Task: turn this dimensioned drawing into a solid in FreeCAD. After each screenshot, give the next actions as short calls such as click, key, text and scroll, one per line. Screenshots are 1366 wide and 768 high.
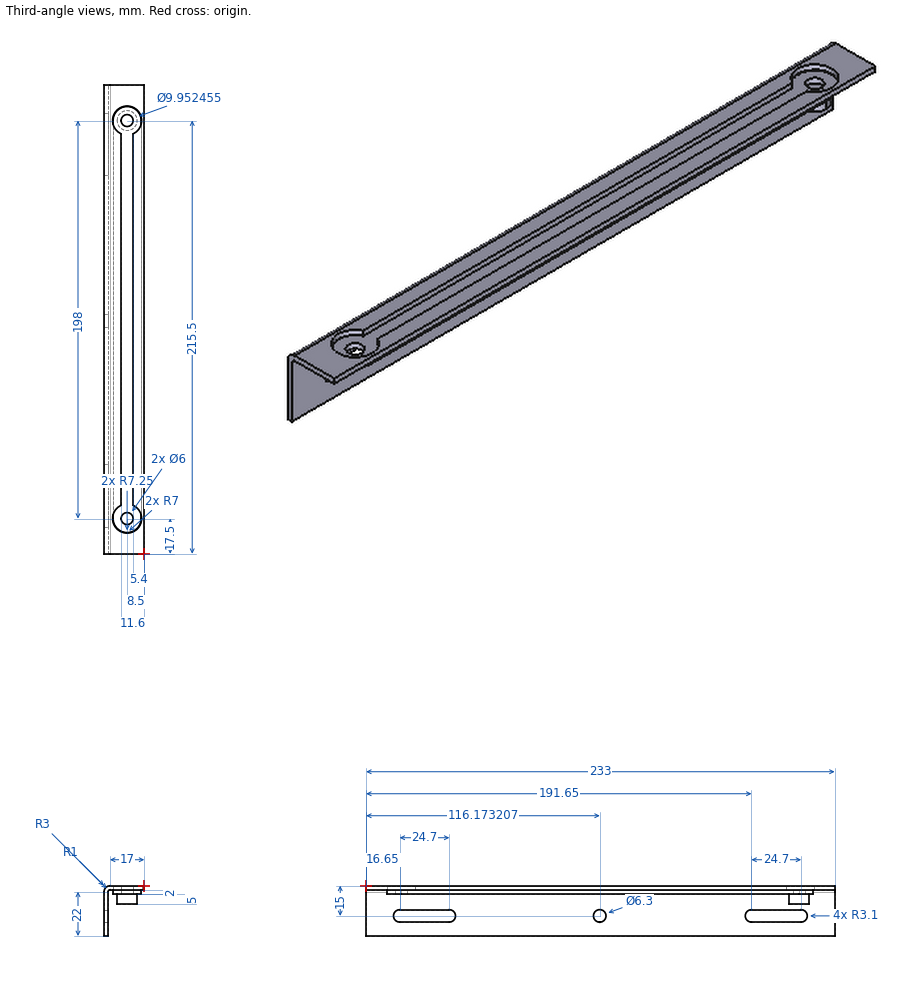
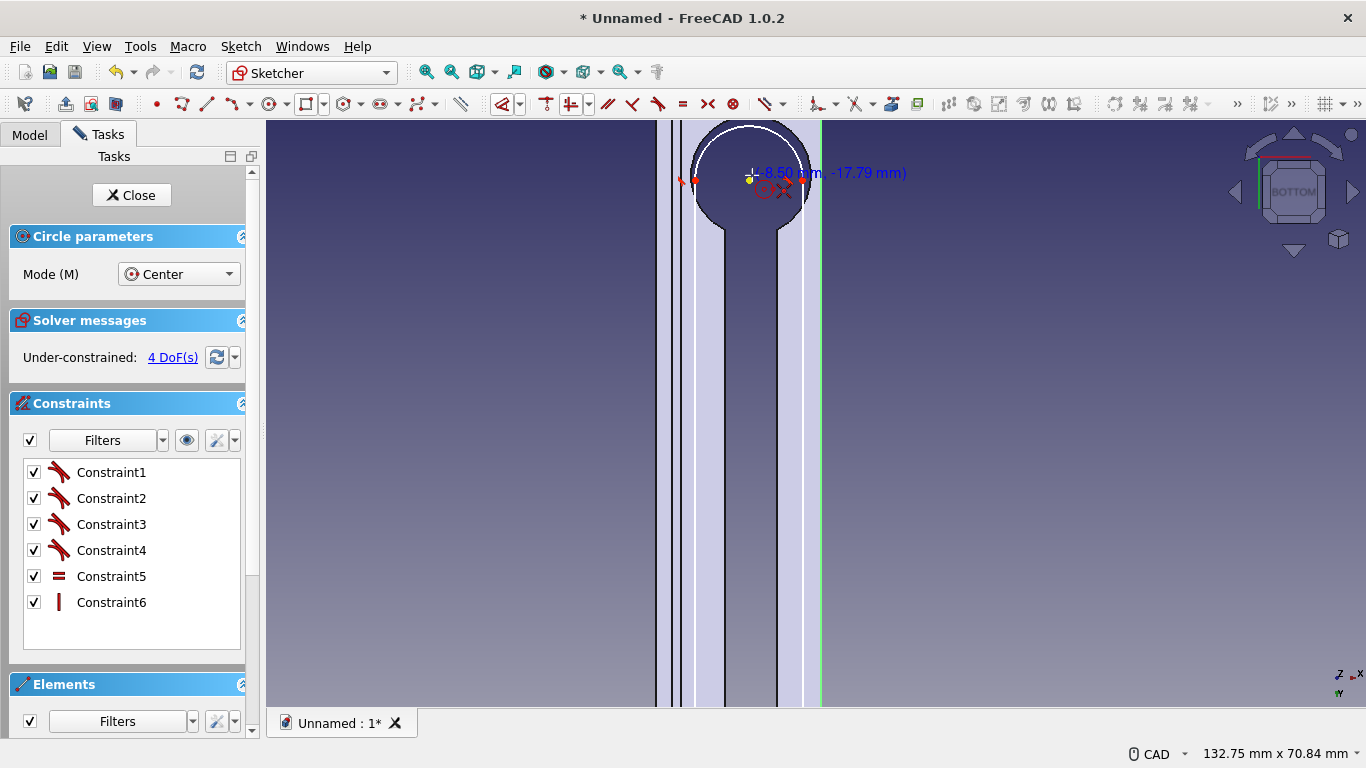
scroll(745, 277, down, 8)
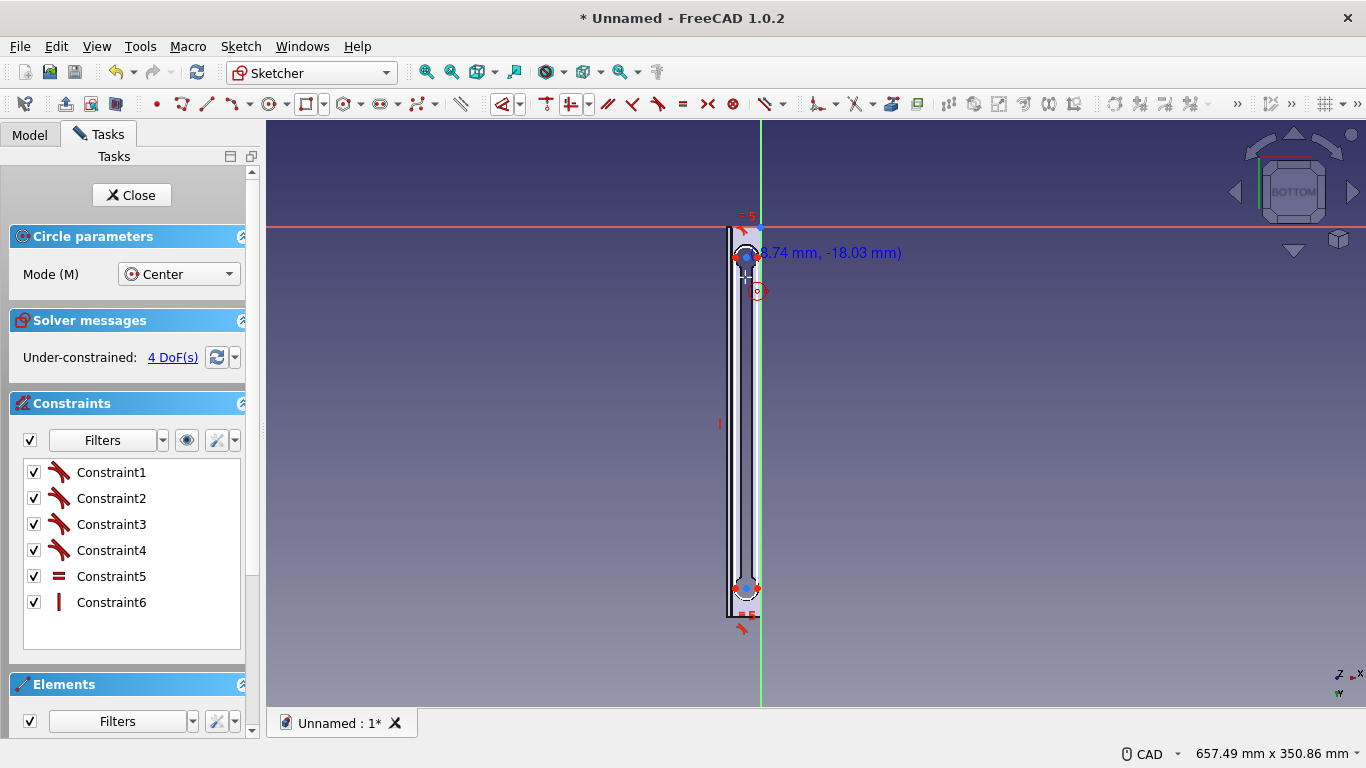
scroll(747, 257, up, 2)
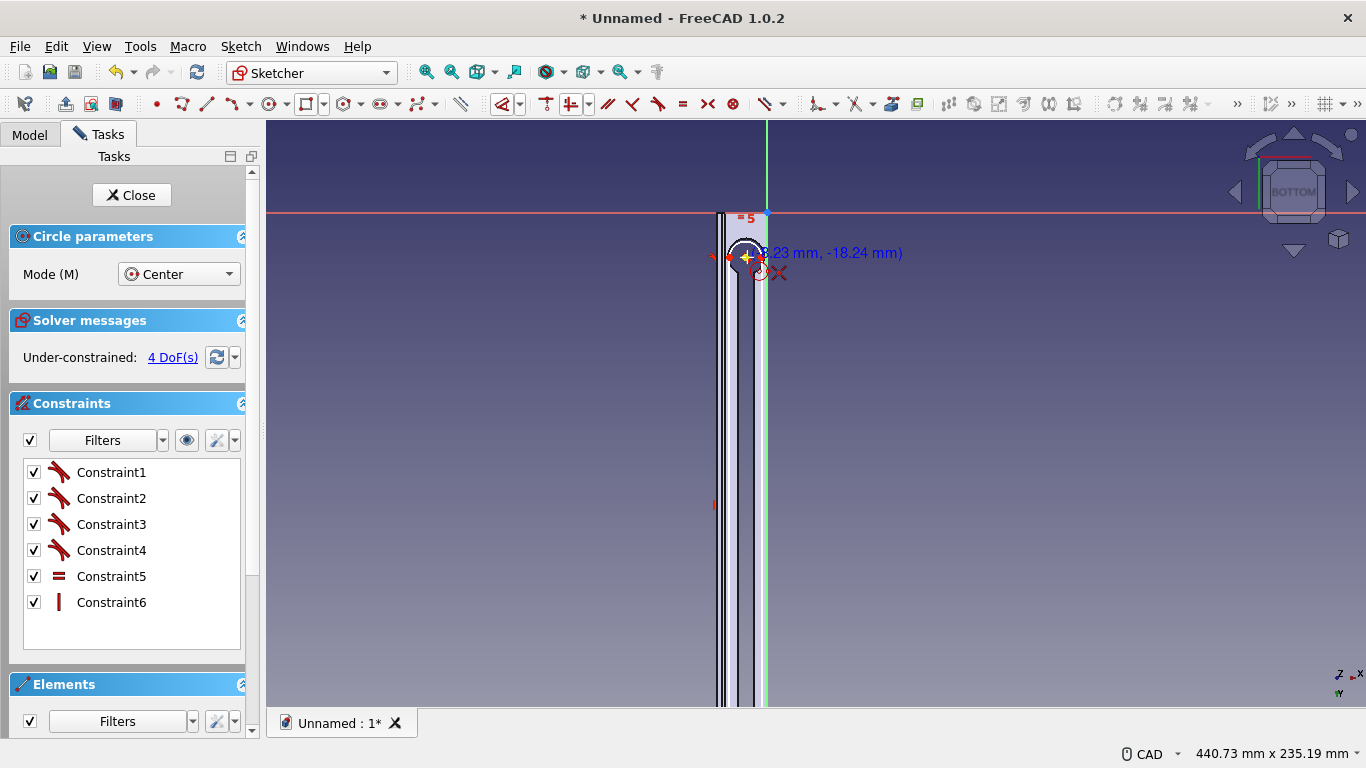
click(746, 258)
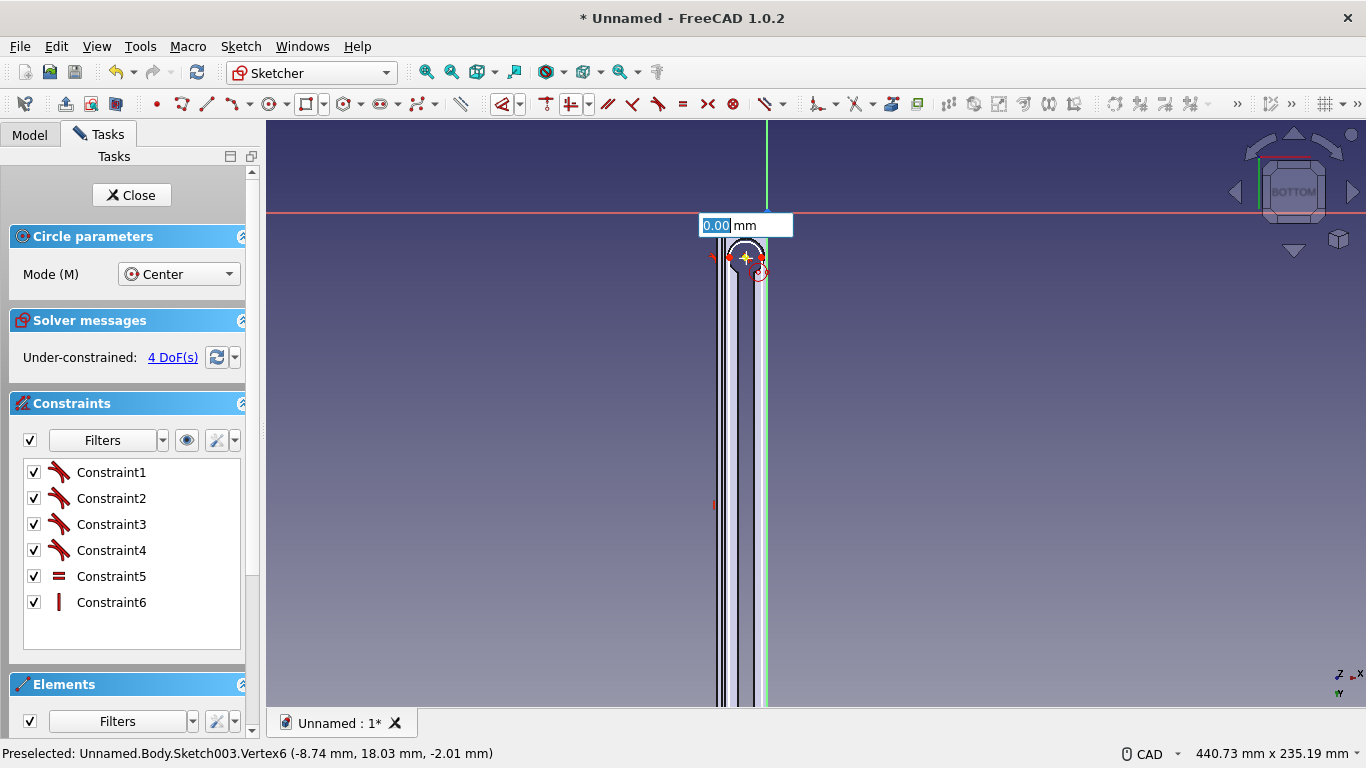
scroll(744, 264, up, 4)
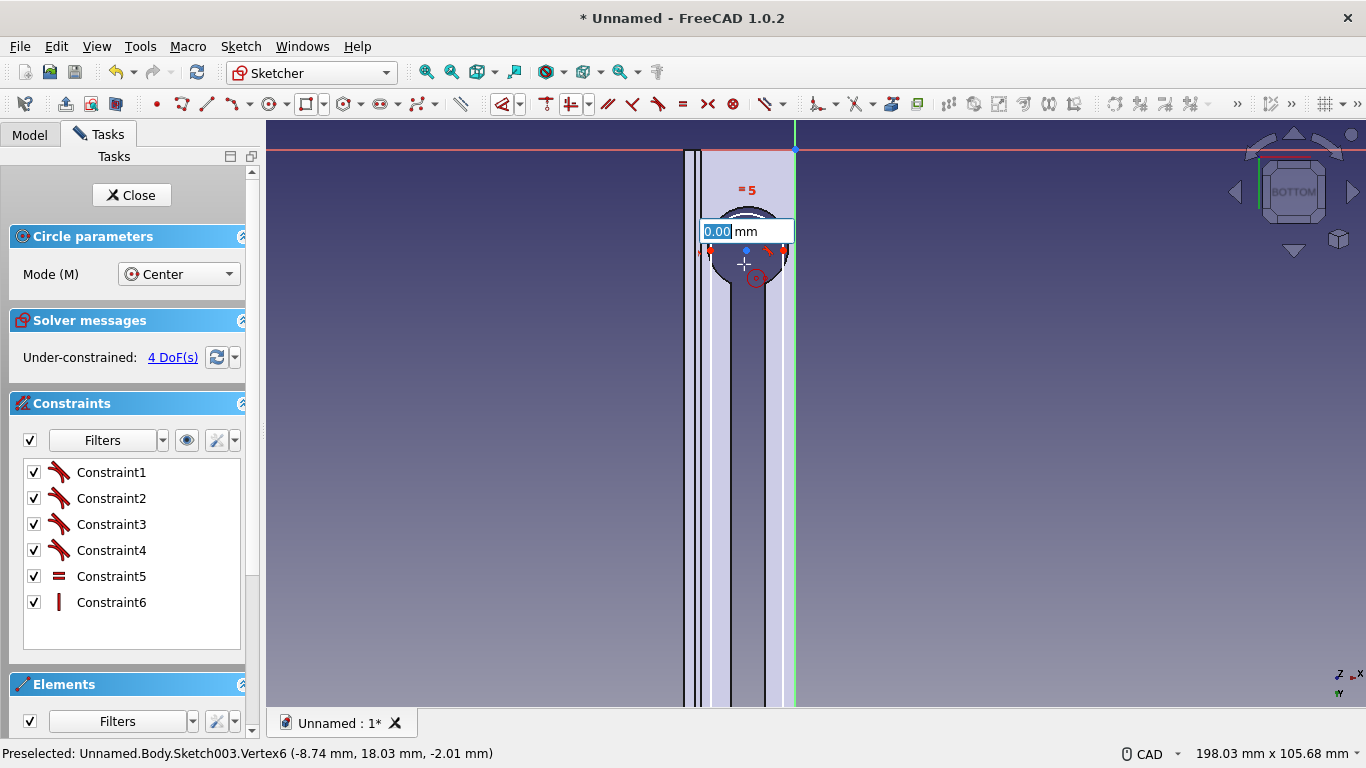
click(742, 263)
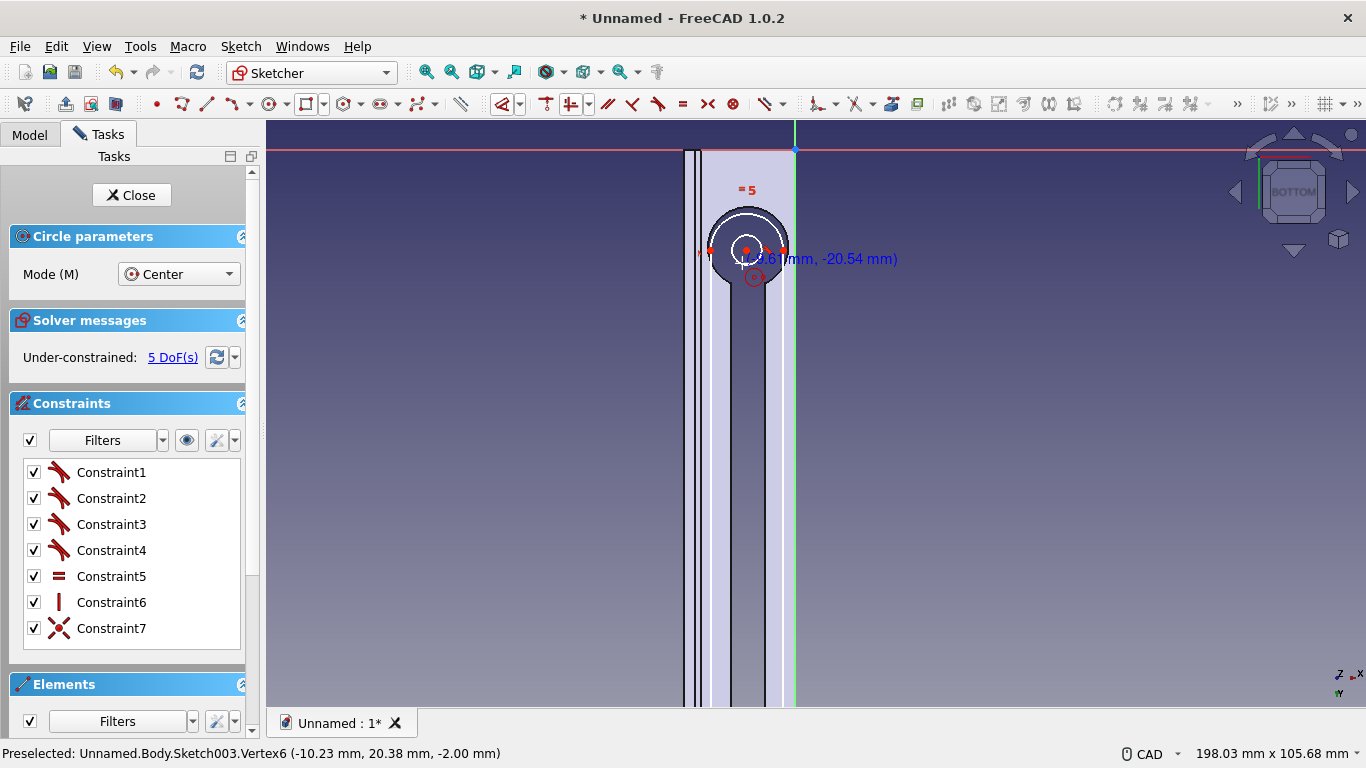
scroll(745, 261, down, 6)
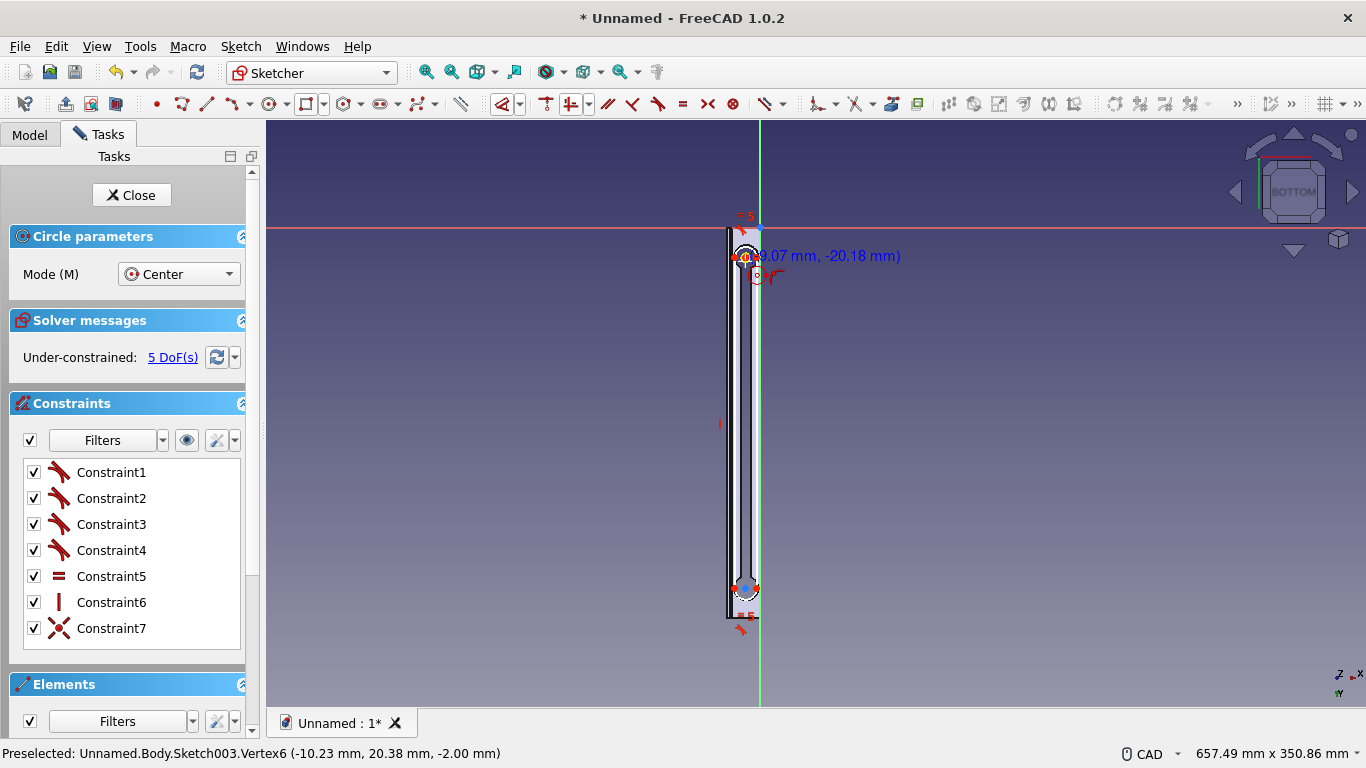
scroll(746, 588, up, 8)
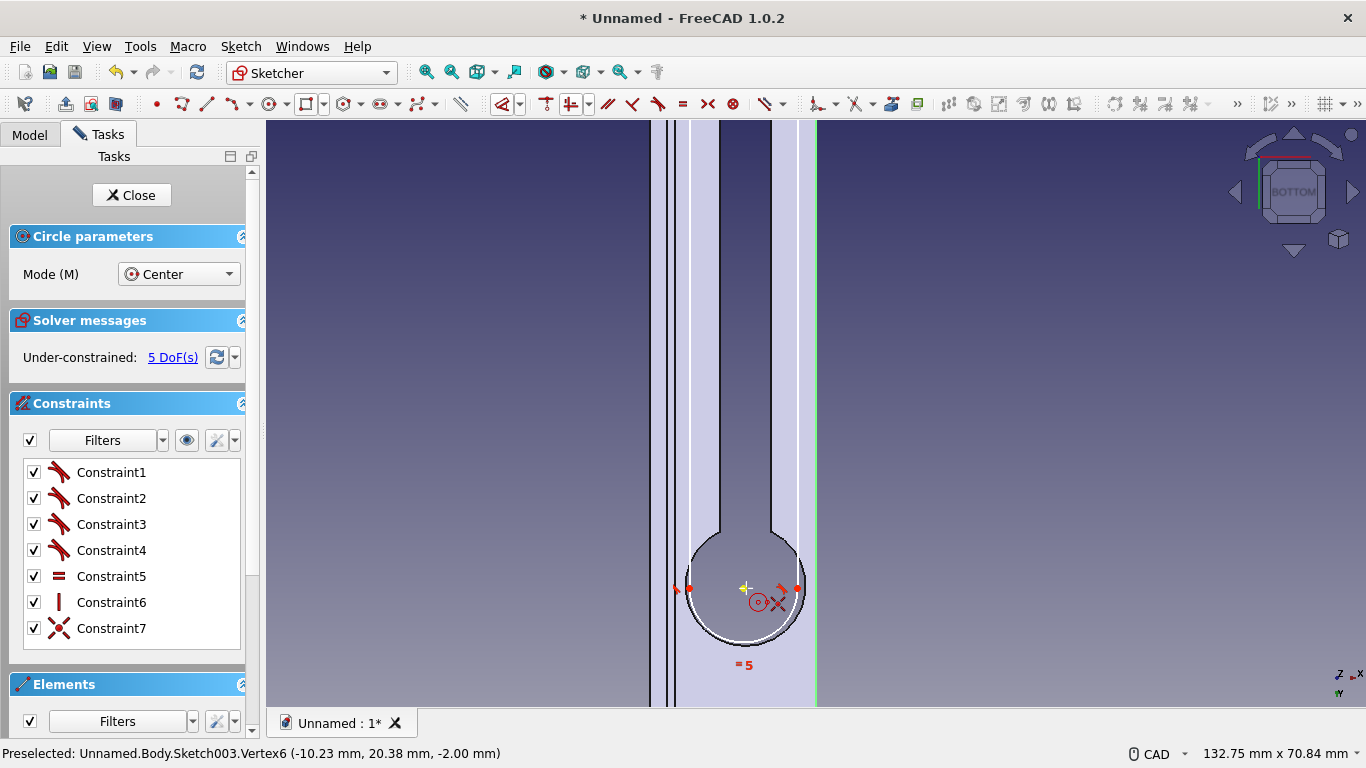
scroll(746, 588, down, 8)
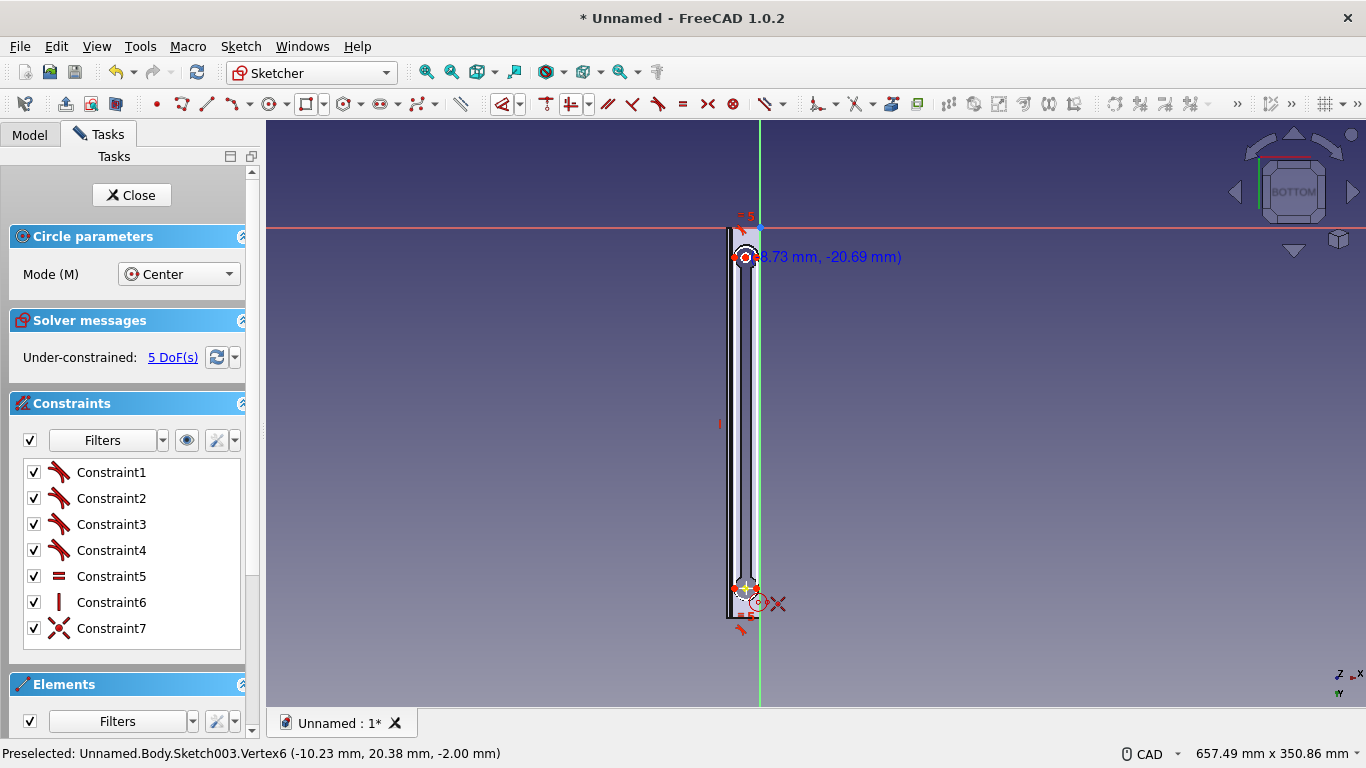
scroll(746, 588, up, 2)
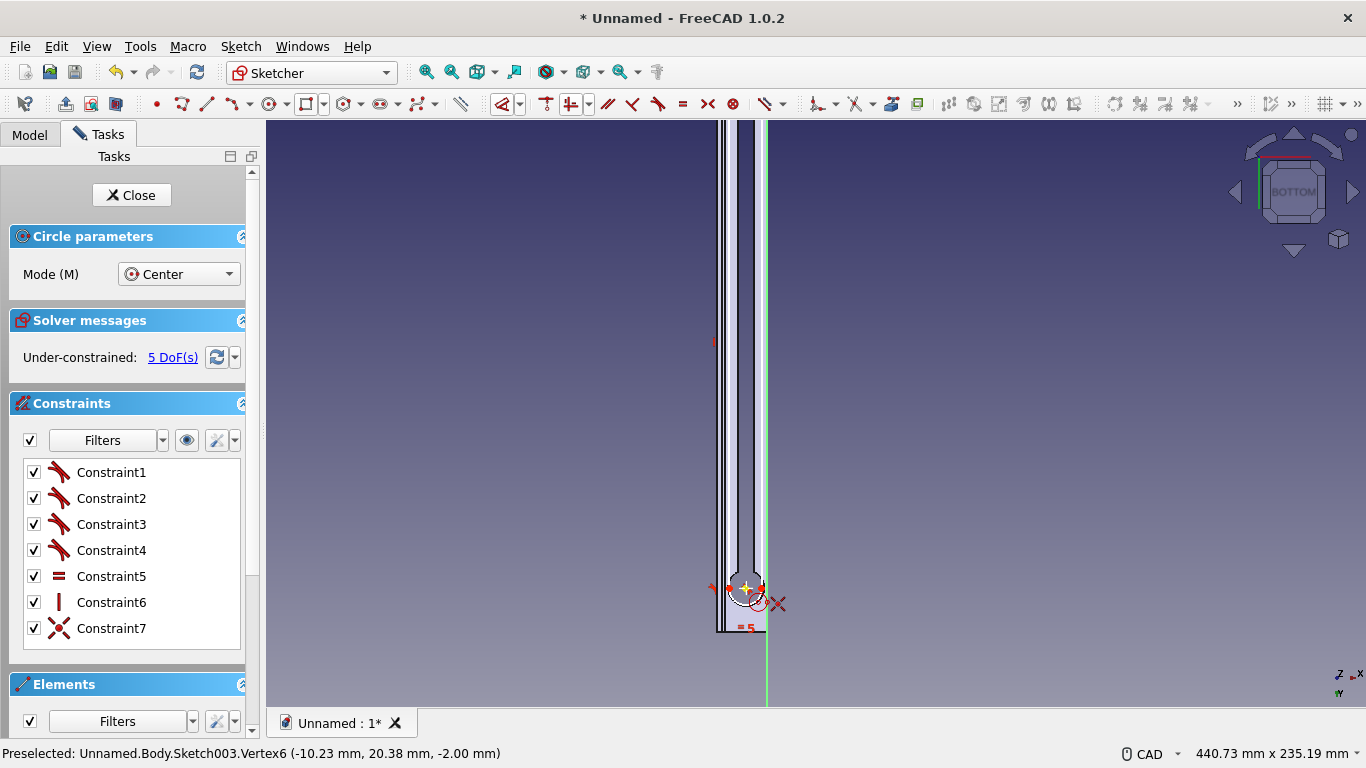
click(746, 589)